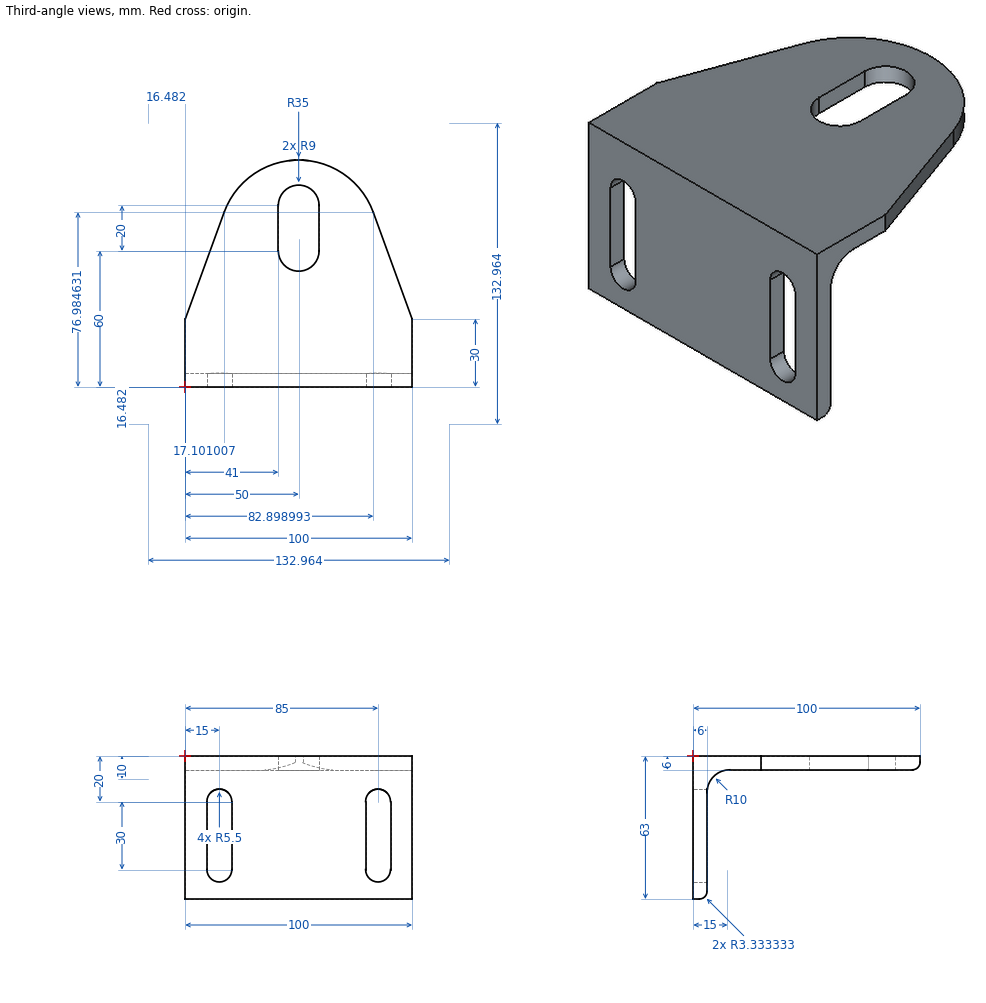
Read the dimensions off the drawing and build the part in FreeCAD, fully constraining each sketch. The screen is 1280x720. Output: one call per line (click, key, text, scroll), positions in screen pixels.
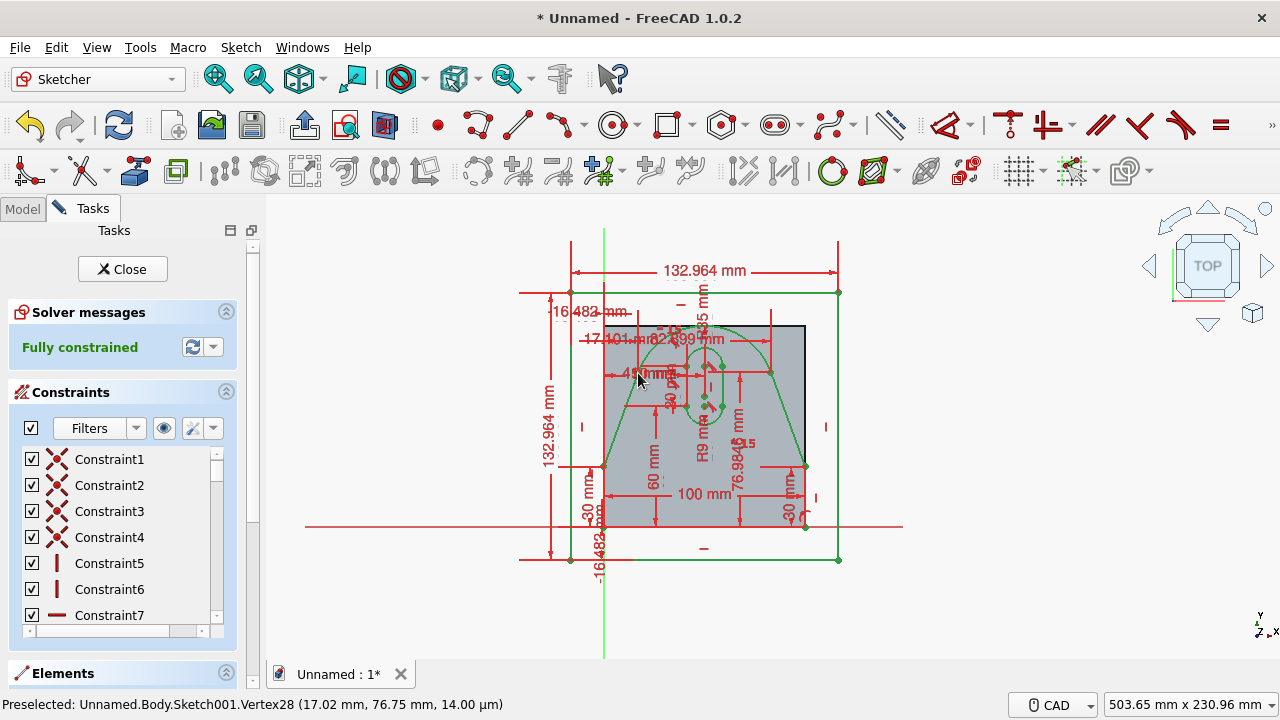
click(123, 269)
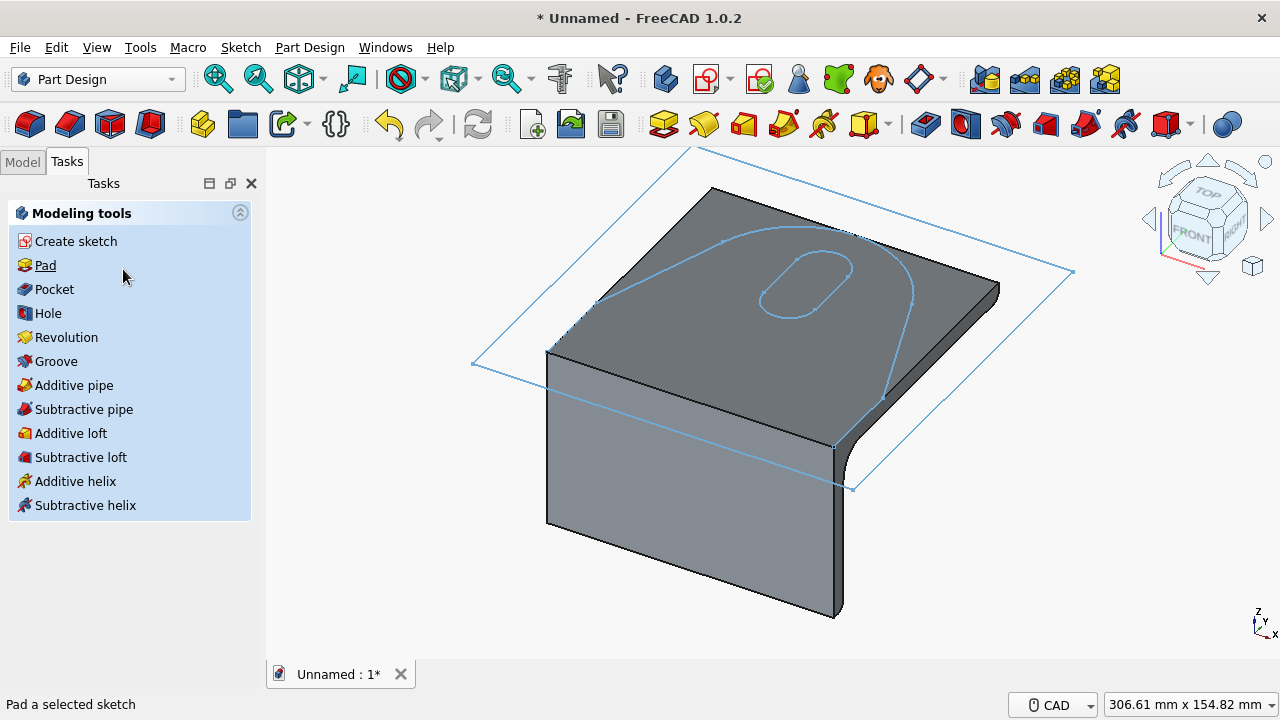
click(926, 124)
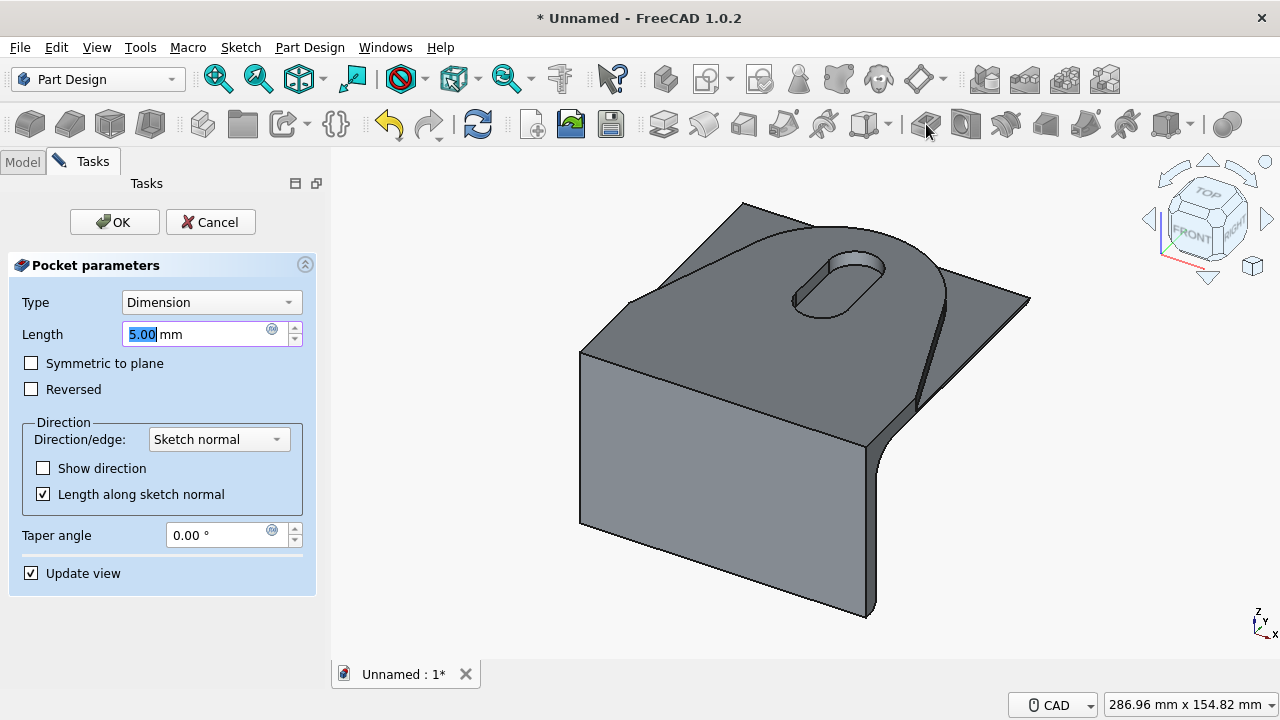
text(10)
key(Tab)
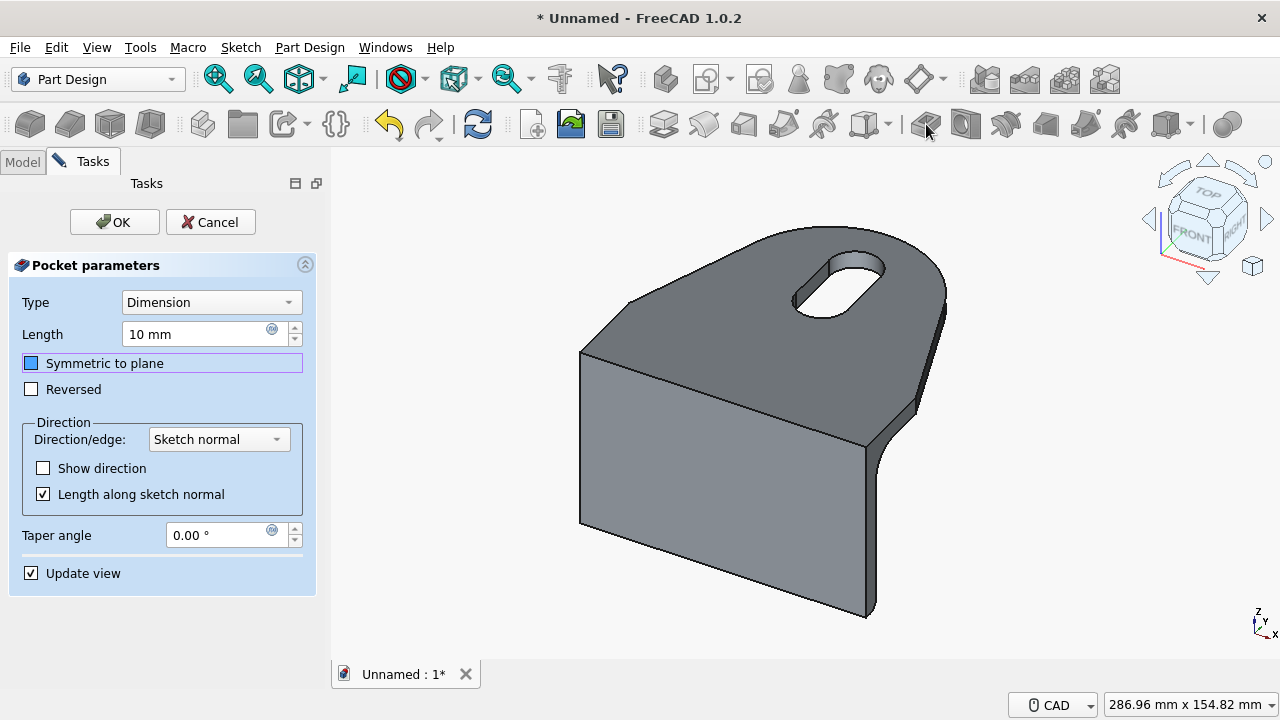
click(115, 222)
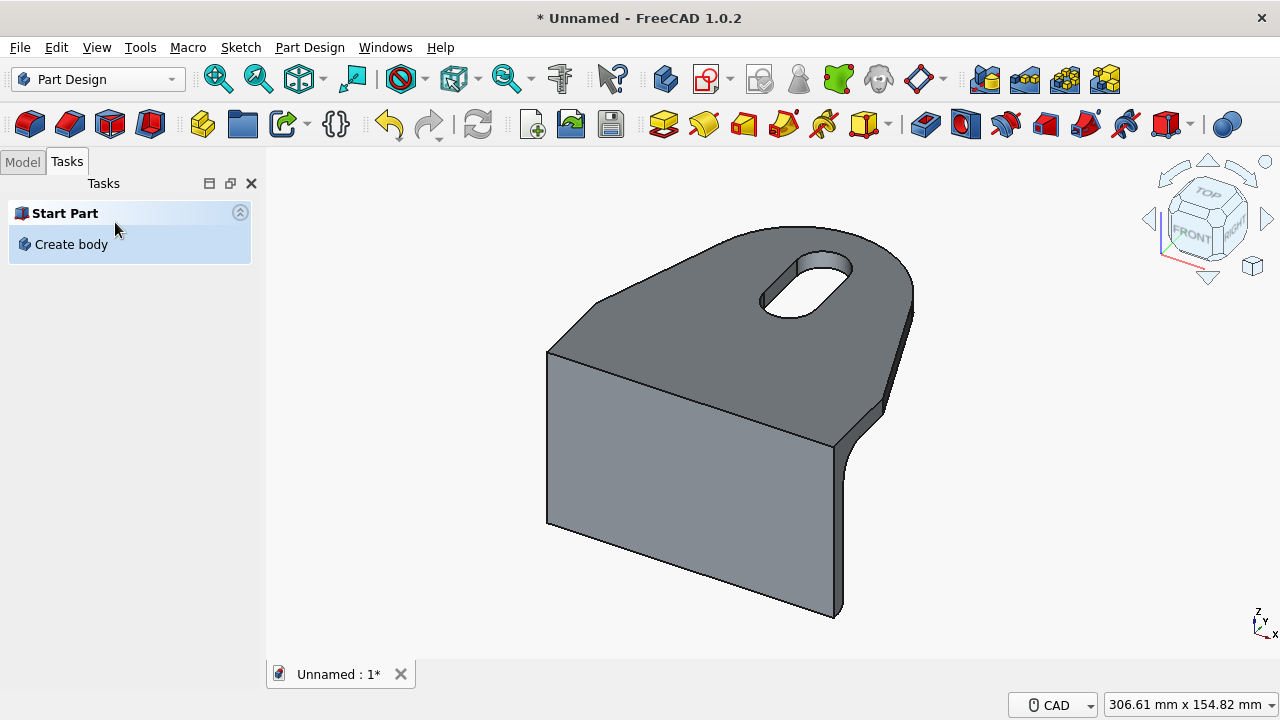
click(649, 471)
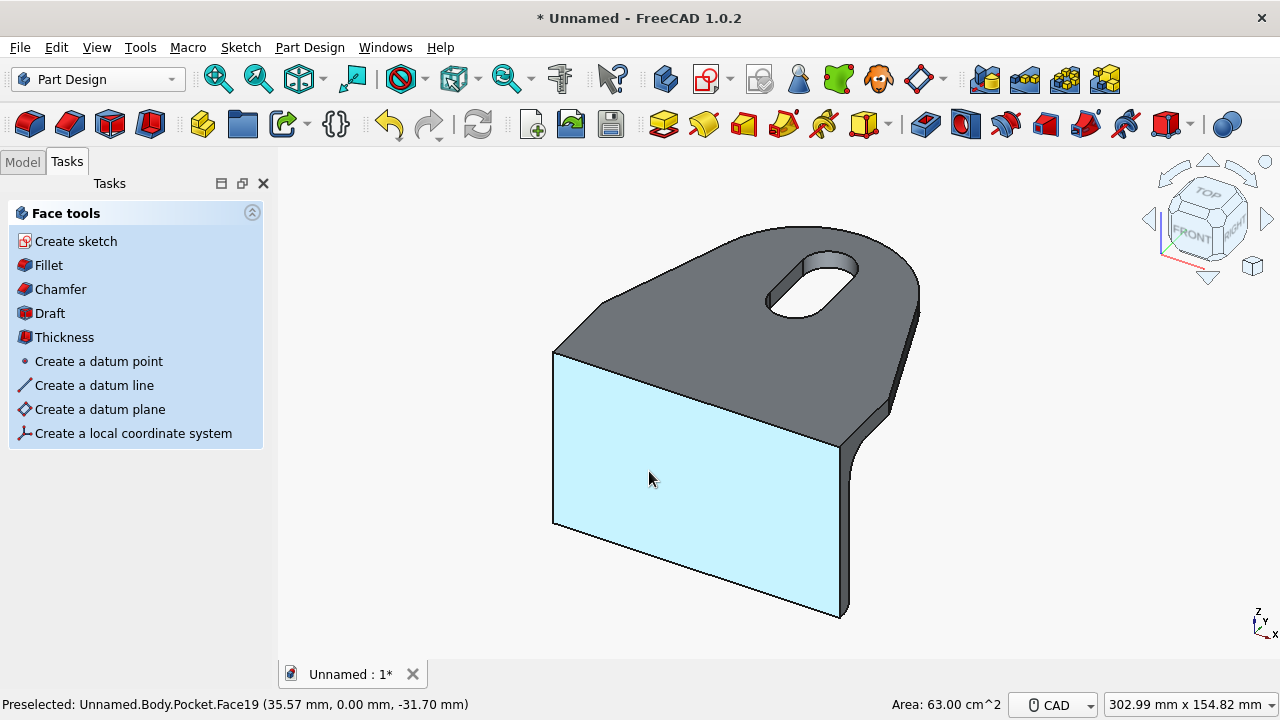
click(706, 80)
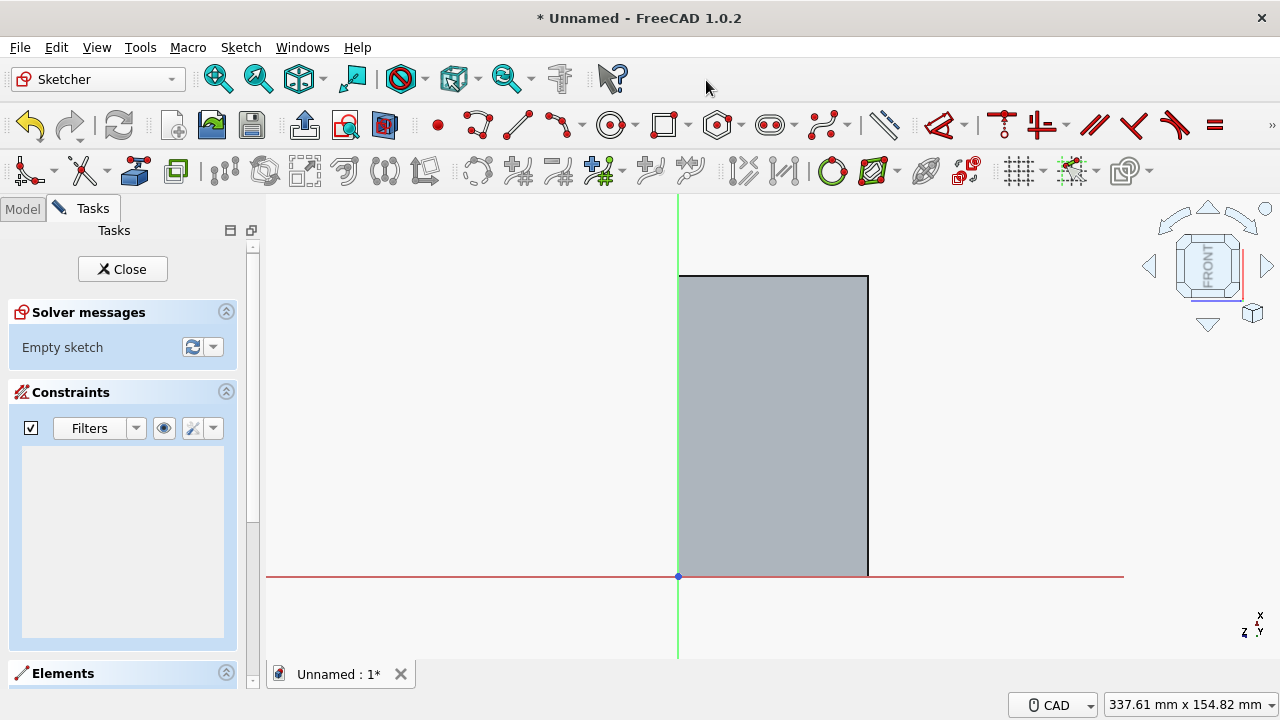
click(770, 126)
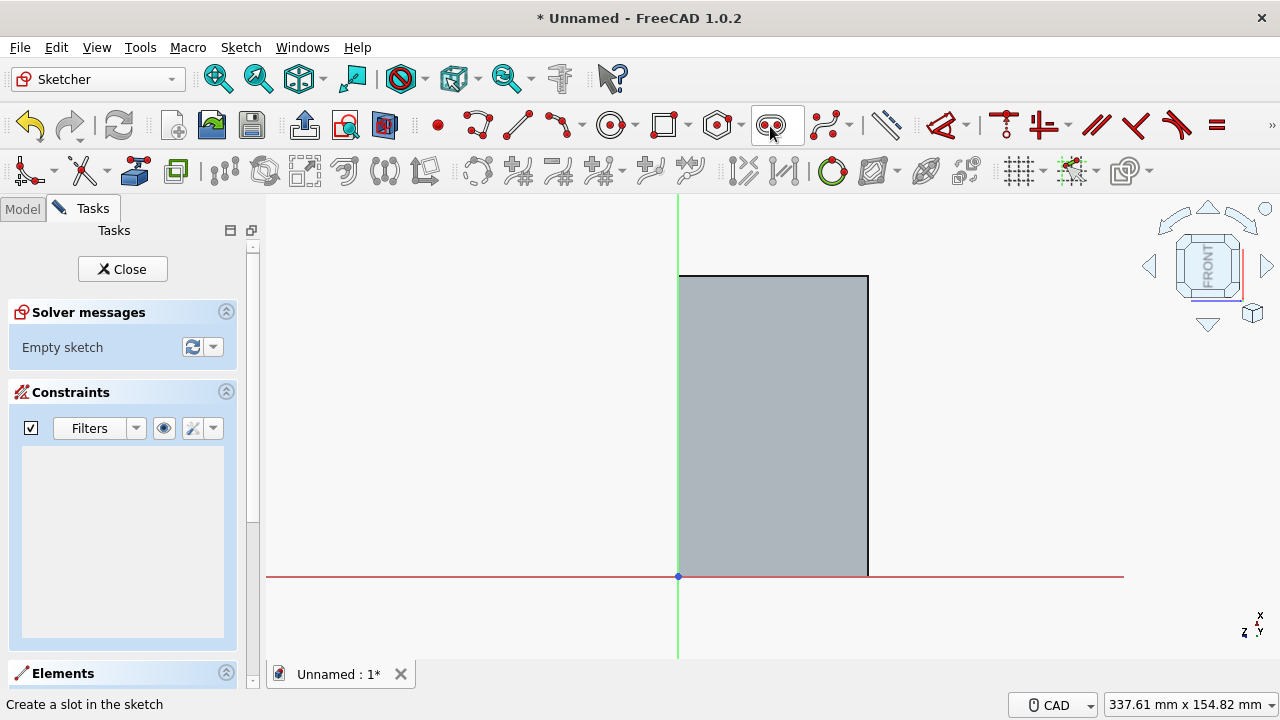
scroll(738, 532, up, 2)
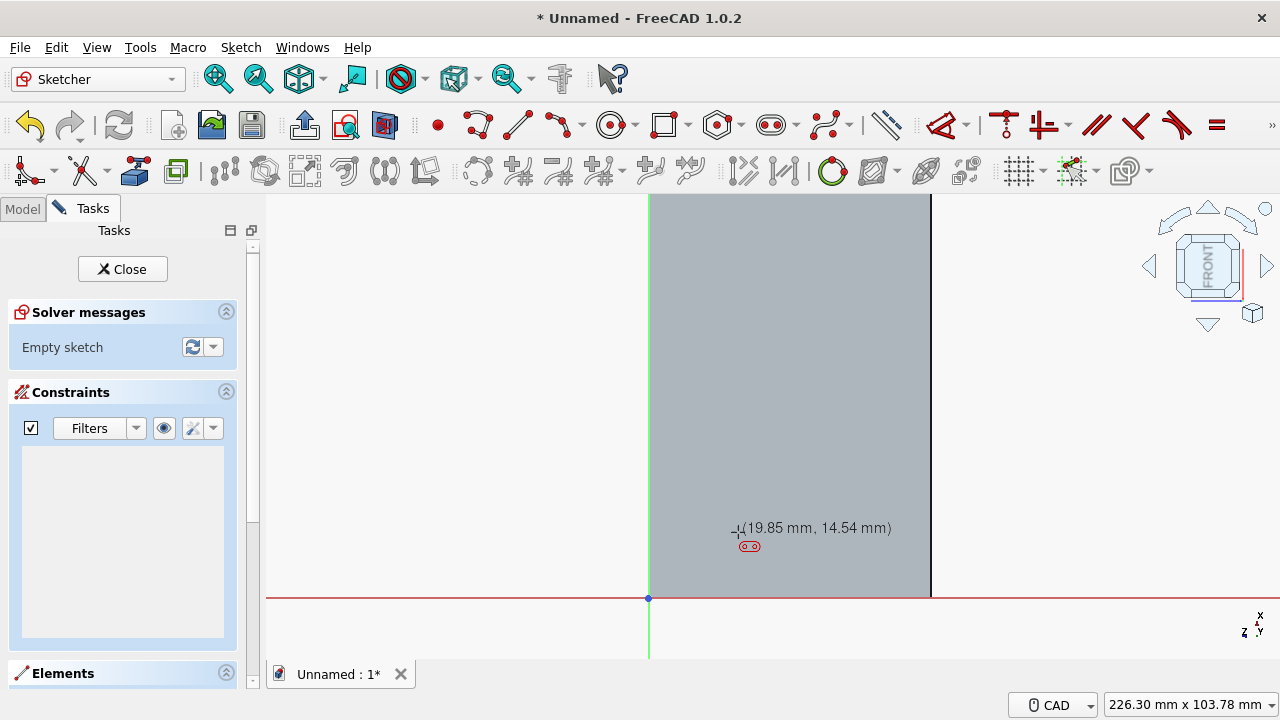
click(738, 531)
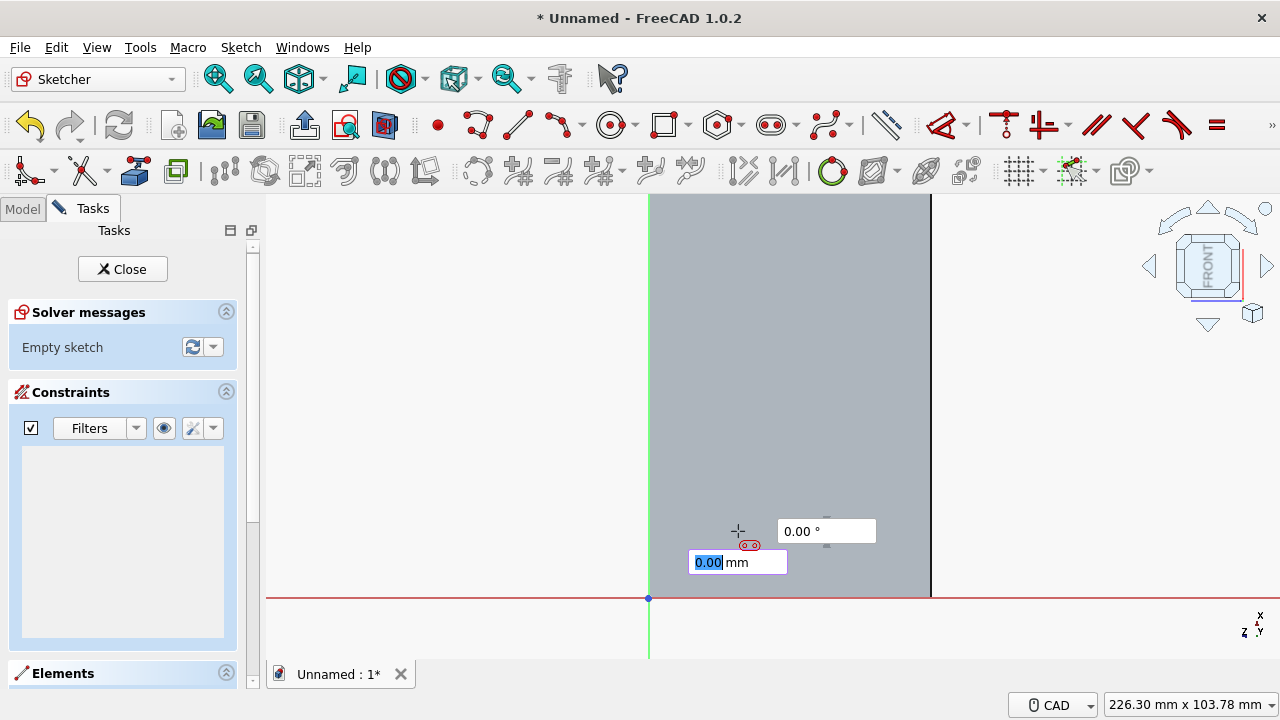
click(873, 531)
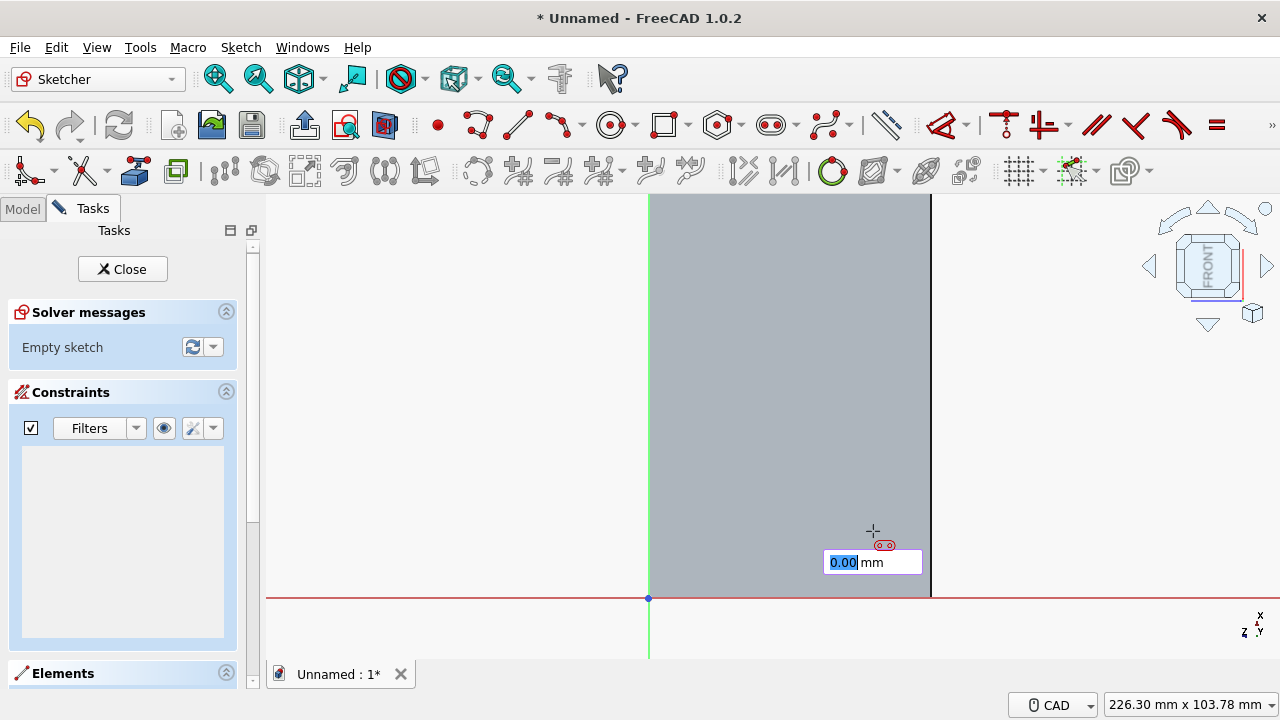
click(806, 506)